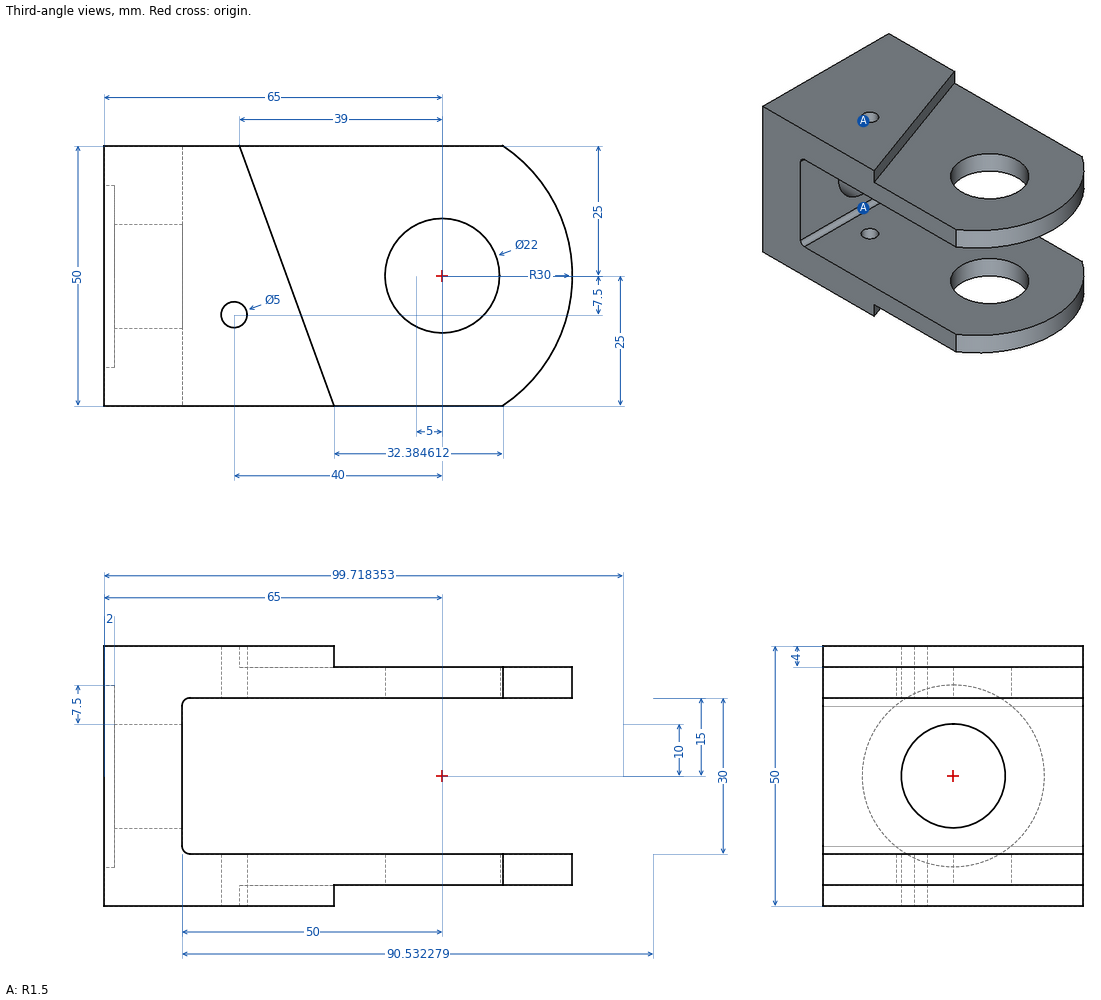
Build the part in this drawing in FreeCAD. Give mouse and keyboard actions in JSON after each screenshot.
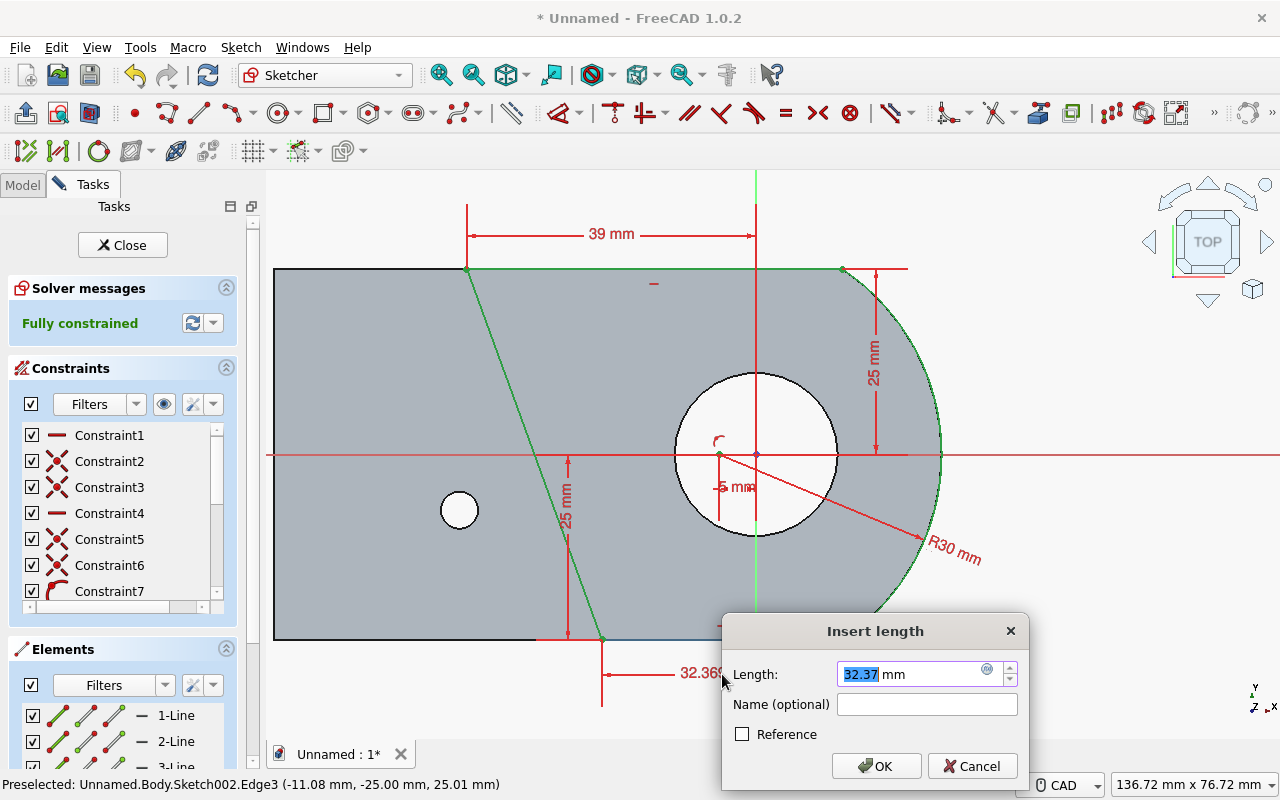
{"action": "type", "text": "32.384612"}
{"action": "key", "text": "Return"}
{"action": "key", "text": "Escape"}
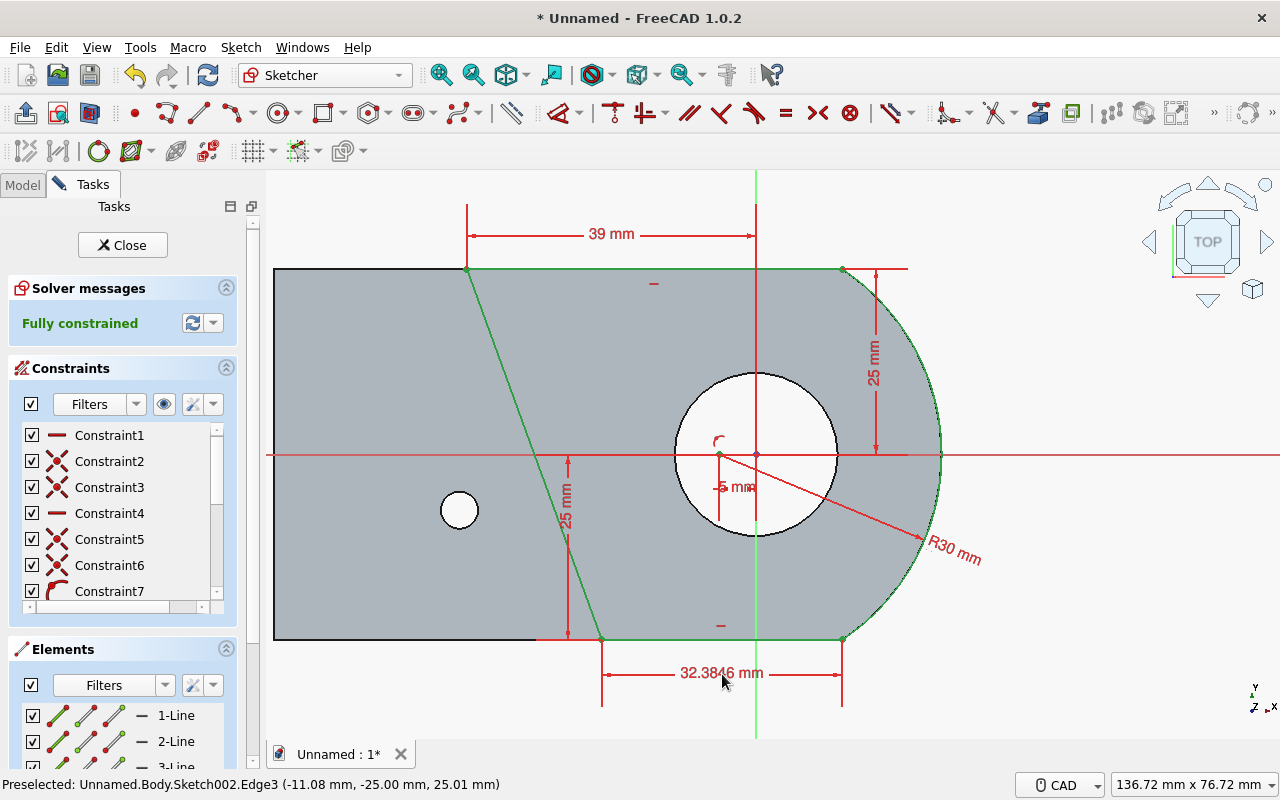
{"action": "left_click", "coordinate": [123, 245]}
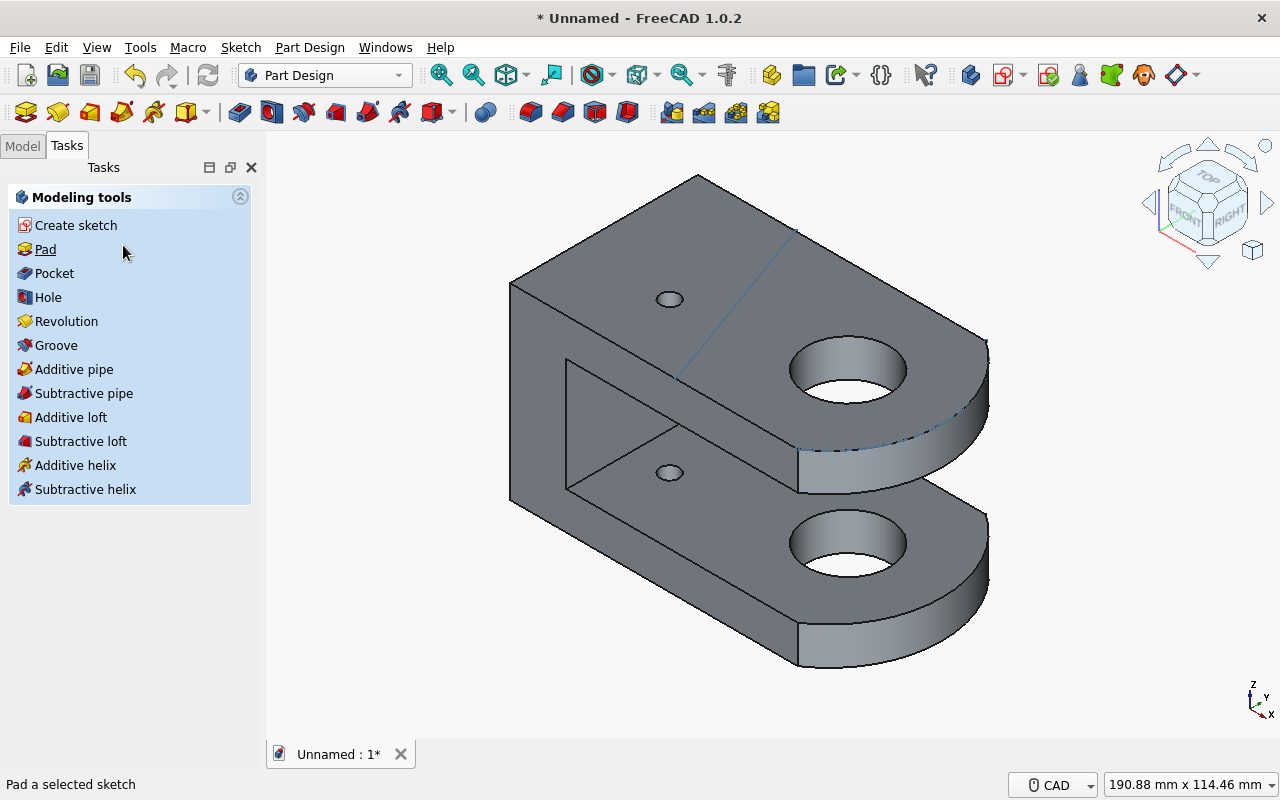
{"action": "left_click", "coordinate": [240, 112]}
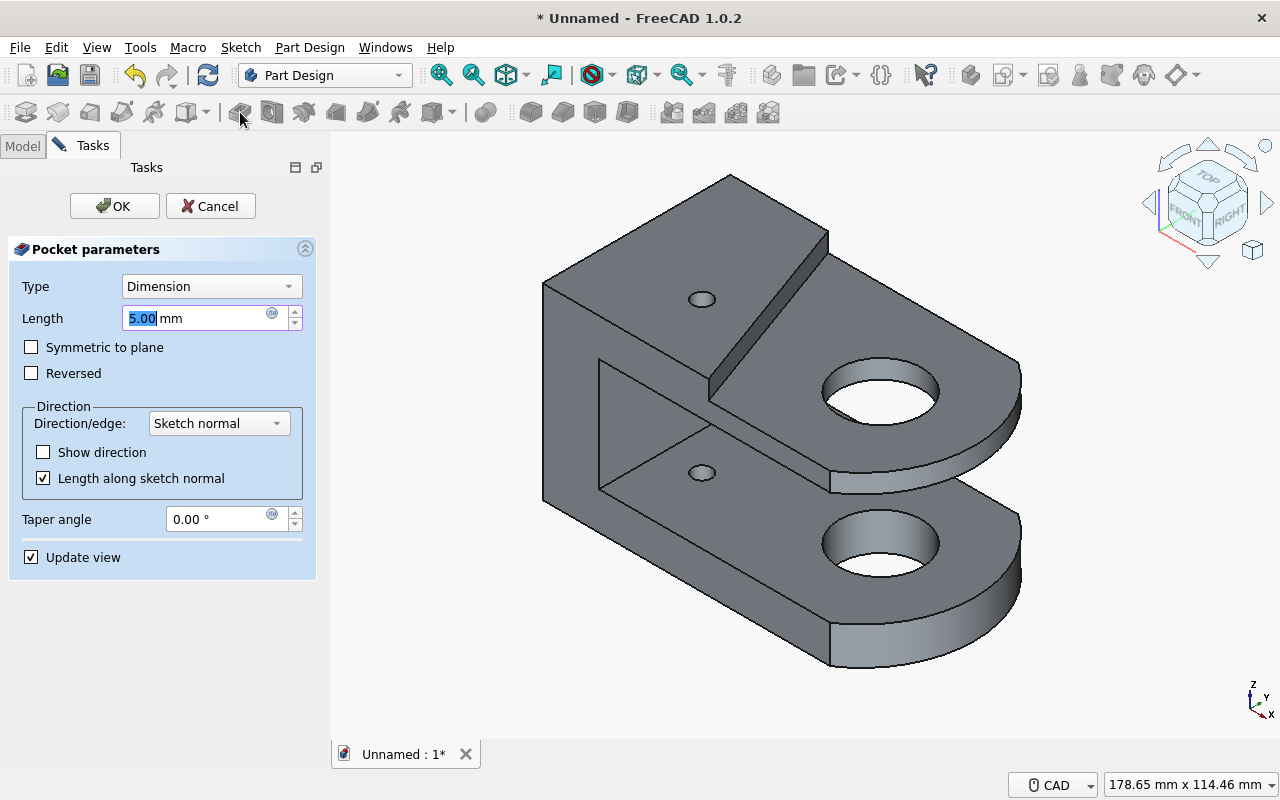
{"action": "type", "text": "4"}
{"action": "key", "text": "Tab"}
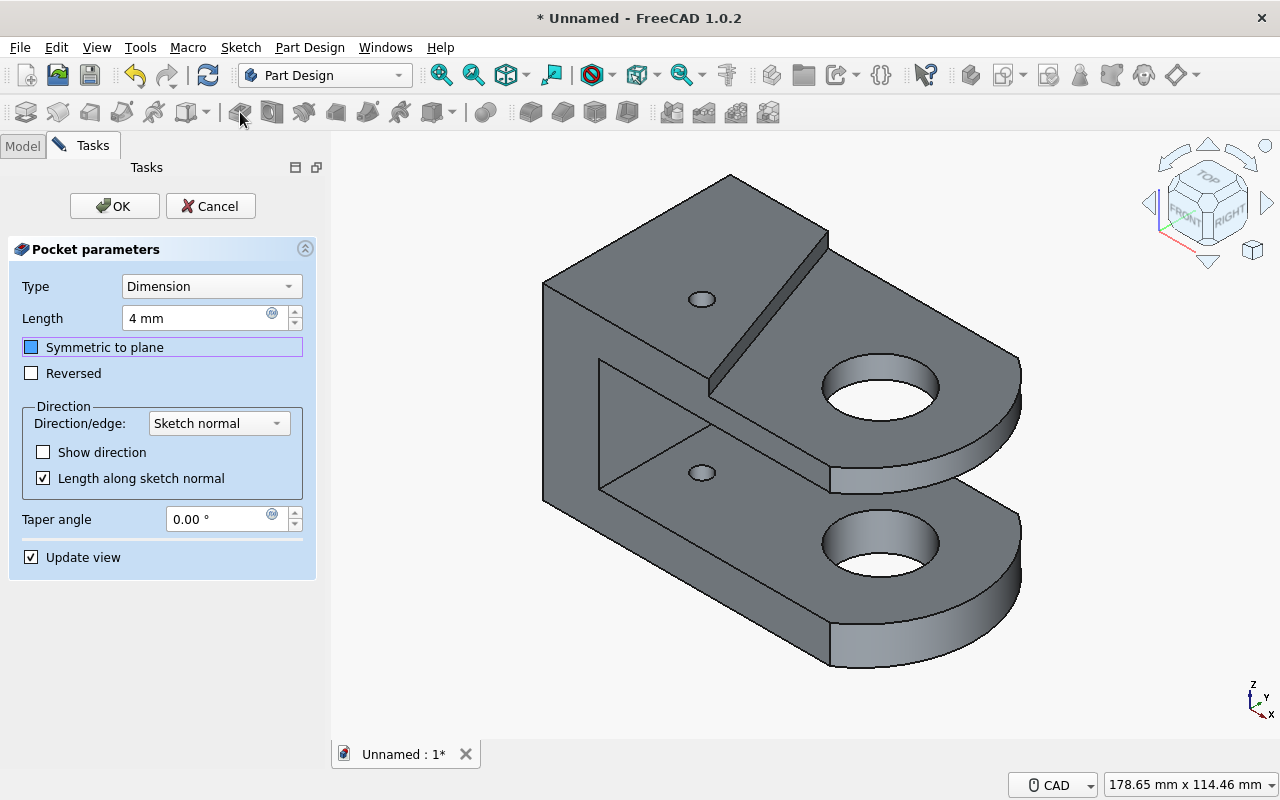
{"action": "left_click", "coordinate": [115, 206]}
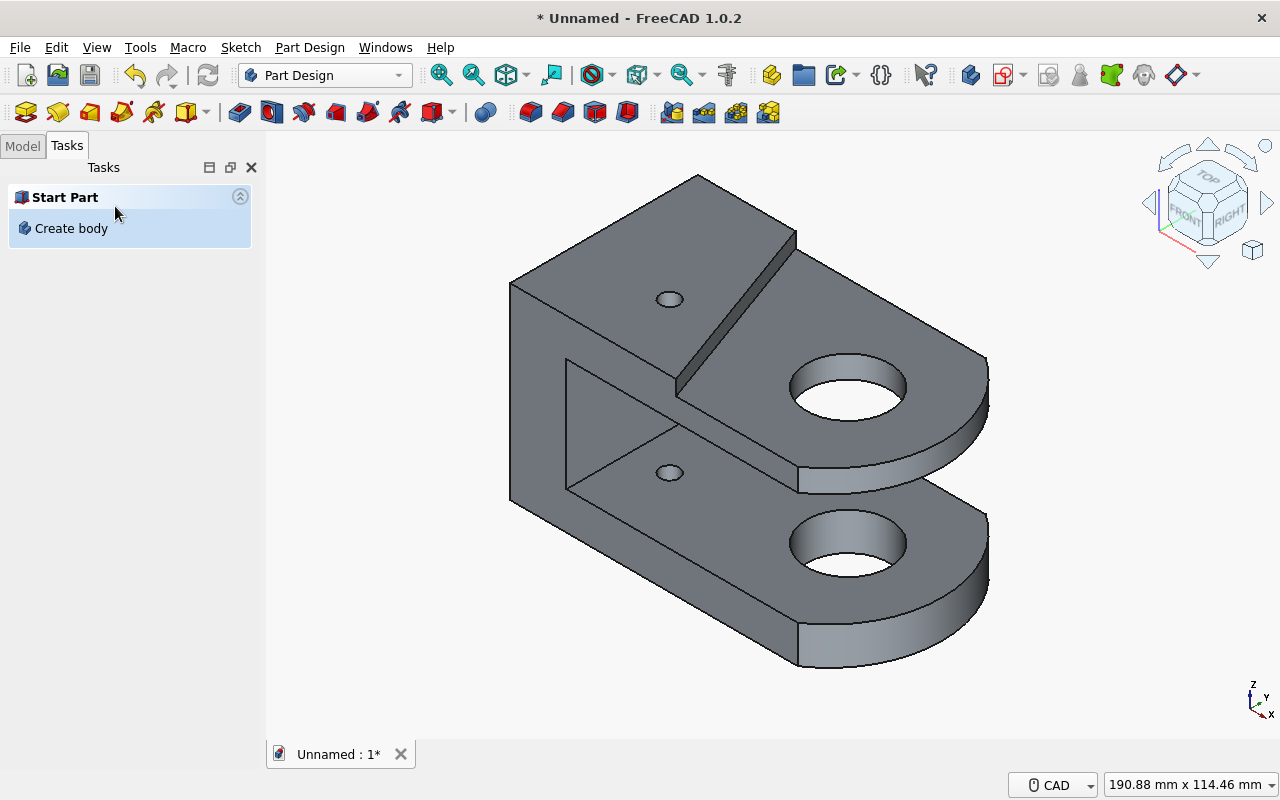
{"action": "left_click", "coordinate": [23, 145]}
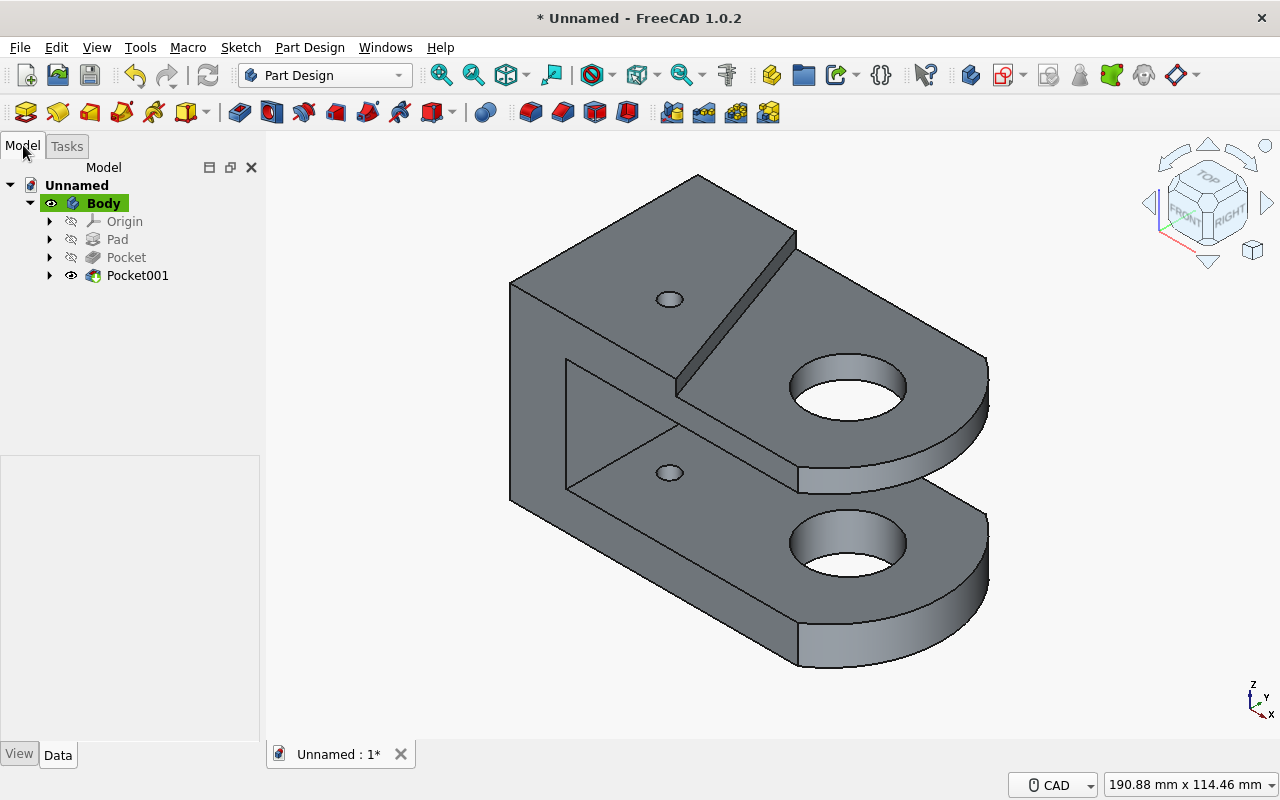
{"action": "left_click", "coordinate": [116, 275]}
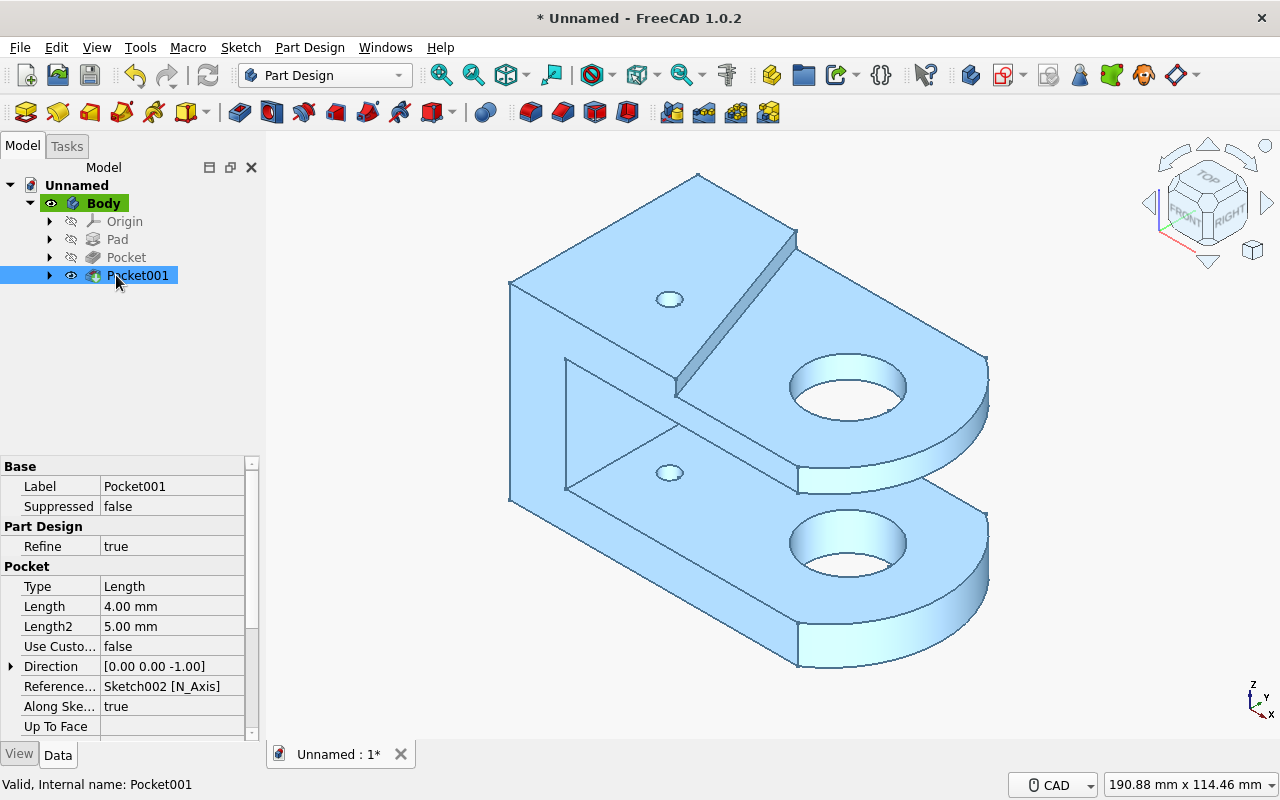
{"action": "left_click", "coordinate": [672, 112]}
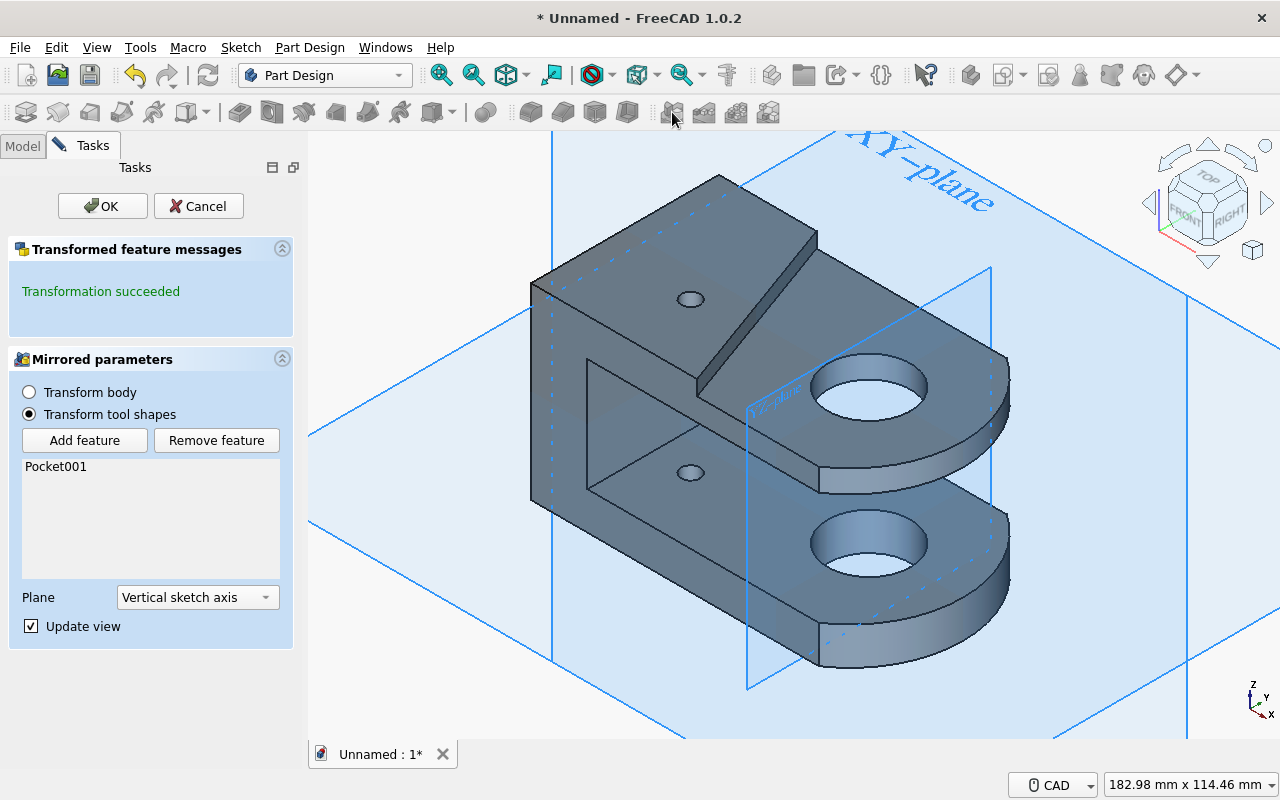
{"action": "left_click", "coordinate": [198, 598]}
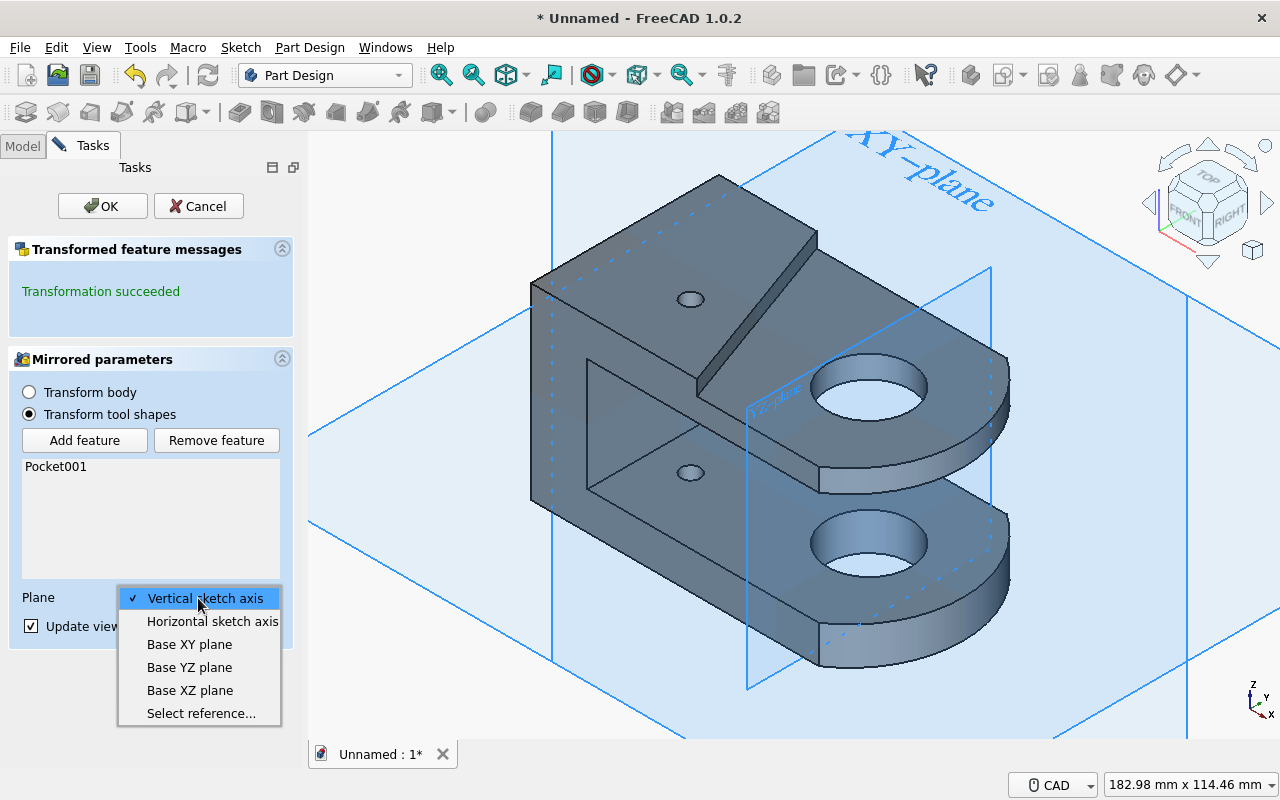
{"action": "left_click", "coordinate": [198, 644]}